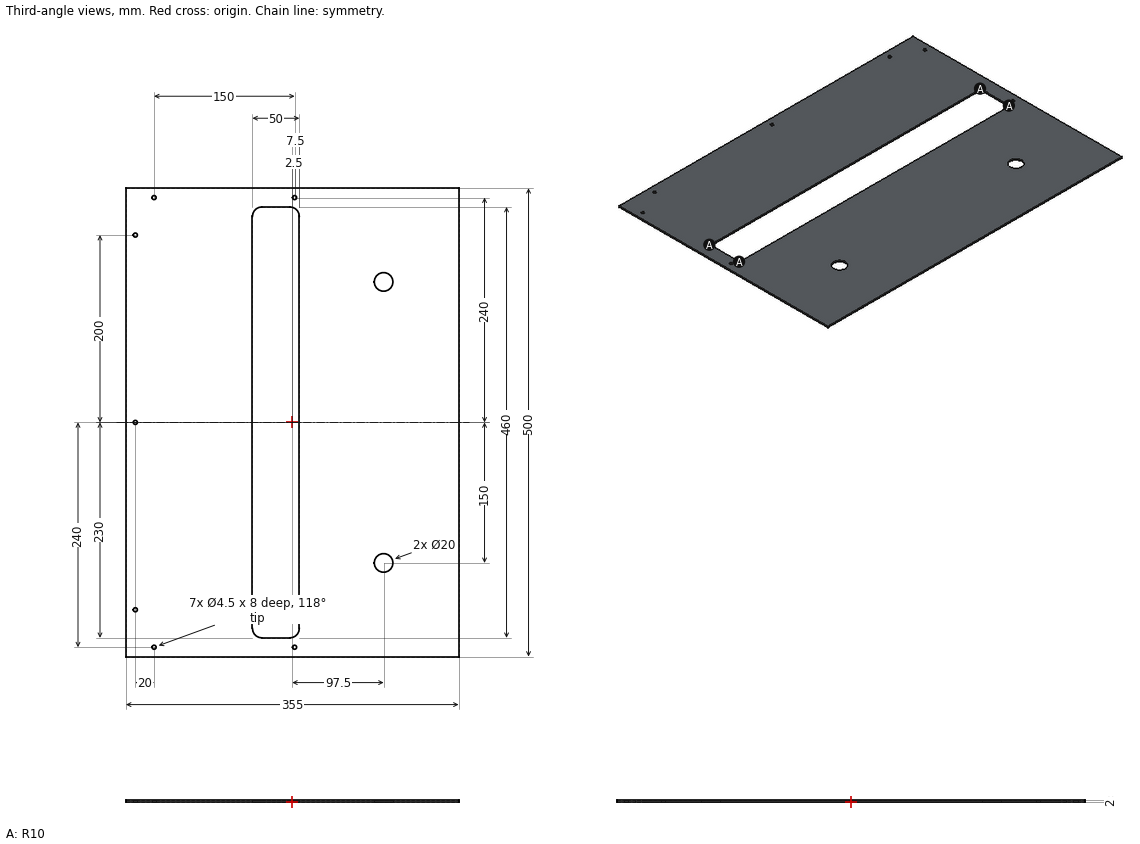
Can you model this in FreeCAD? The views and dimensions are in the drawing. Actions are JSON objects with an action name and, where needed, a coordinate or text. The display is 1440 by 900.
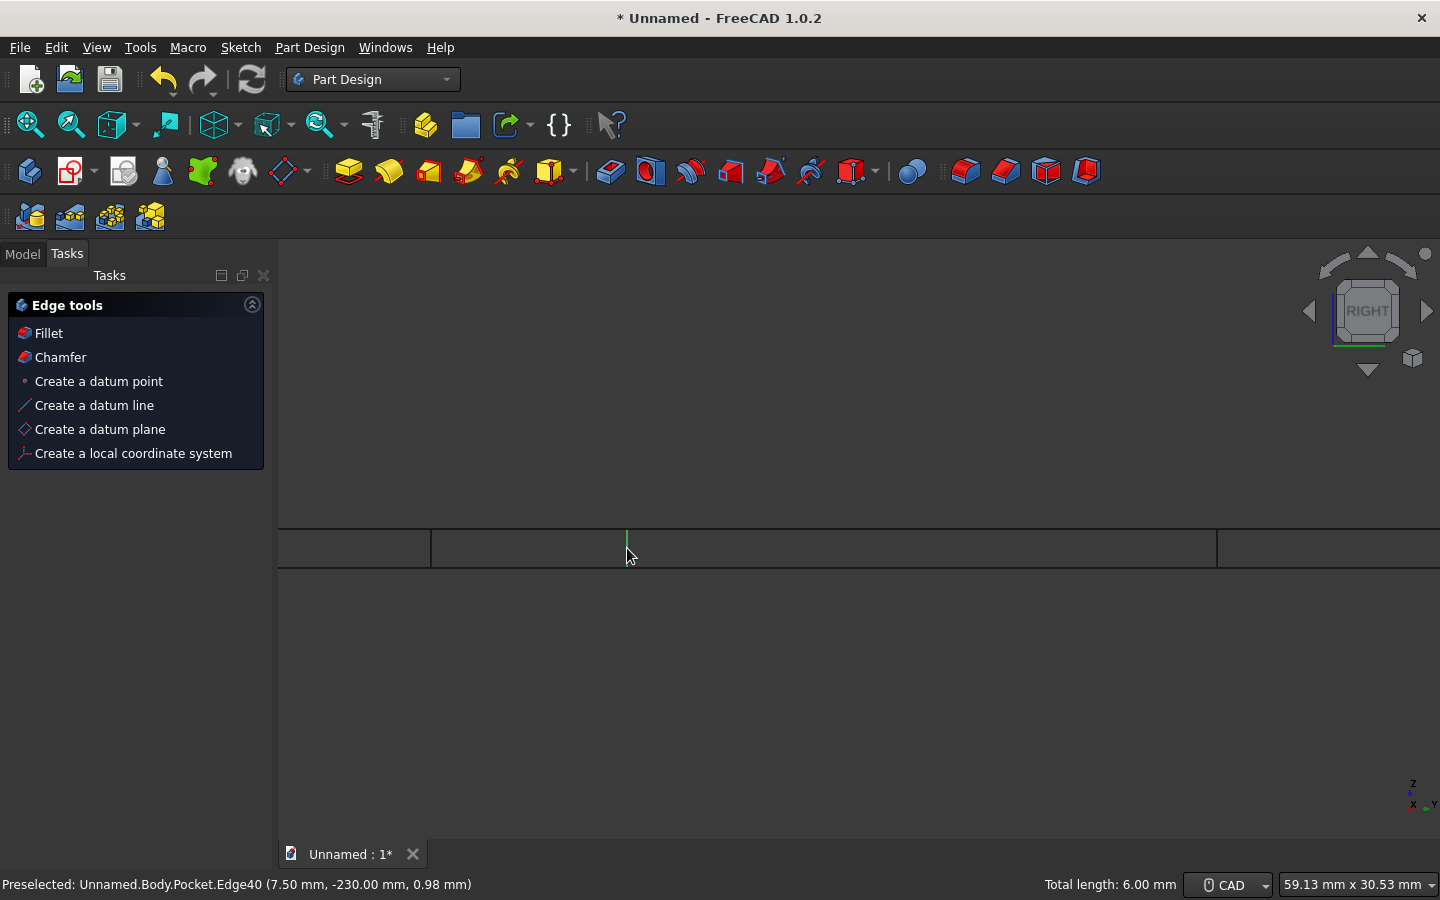
{"action": "left_click", "coordinate": [32, 126]}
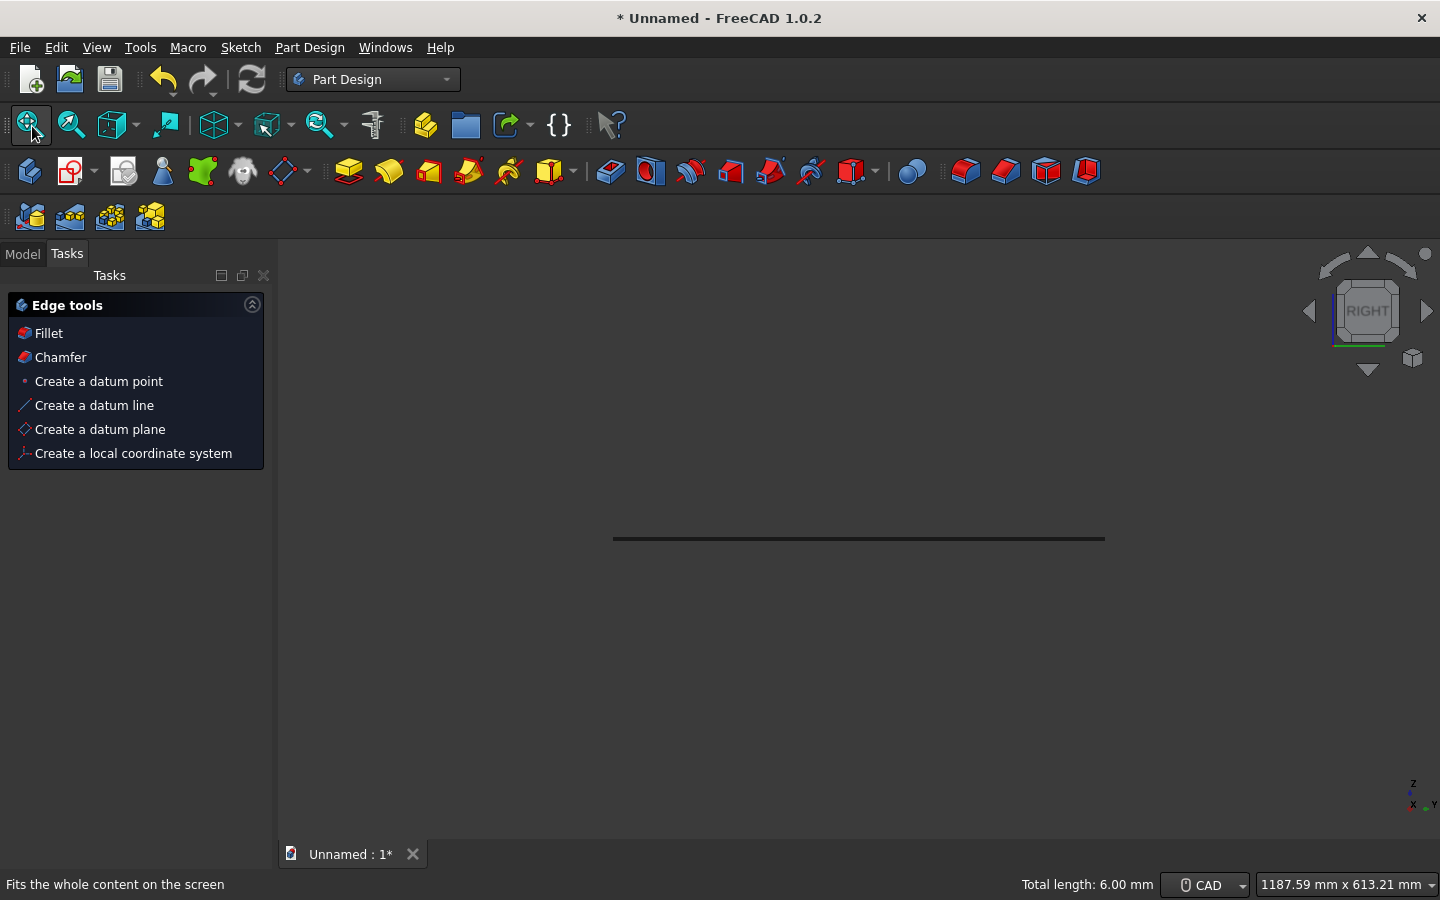
{"action": "key", "text": "5"}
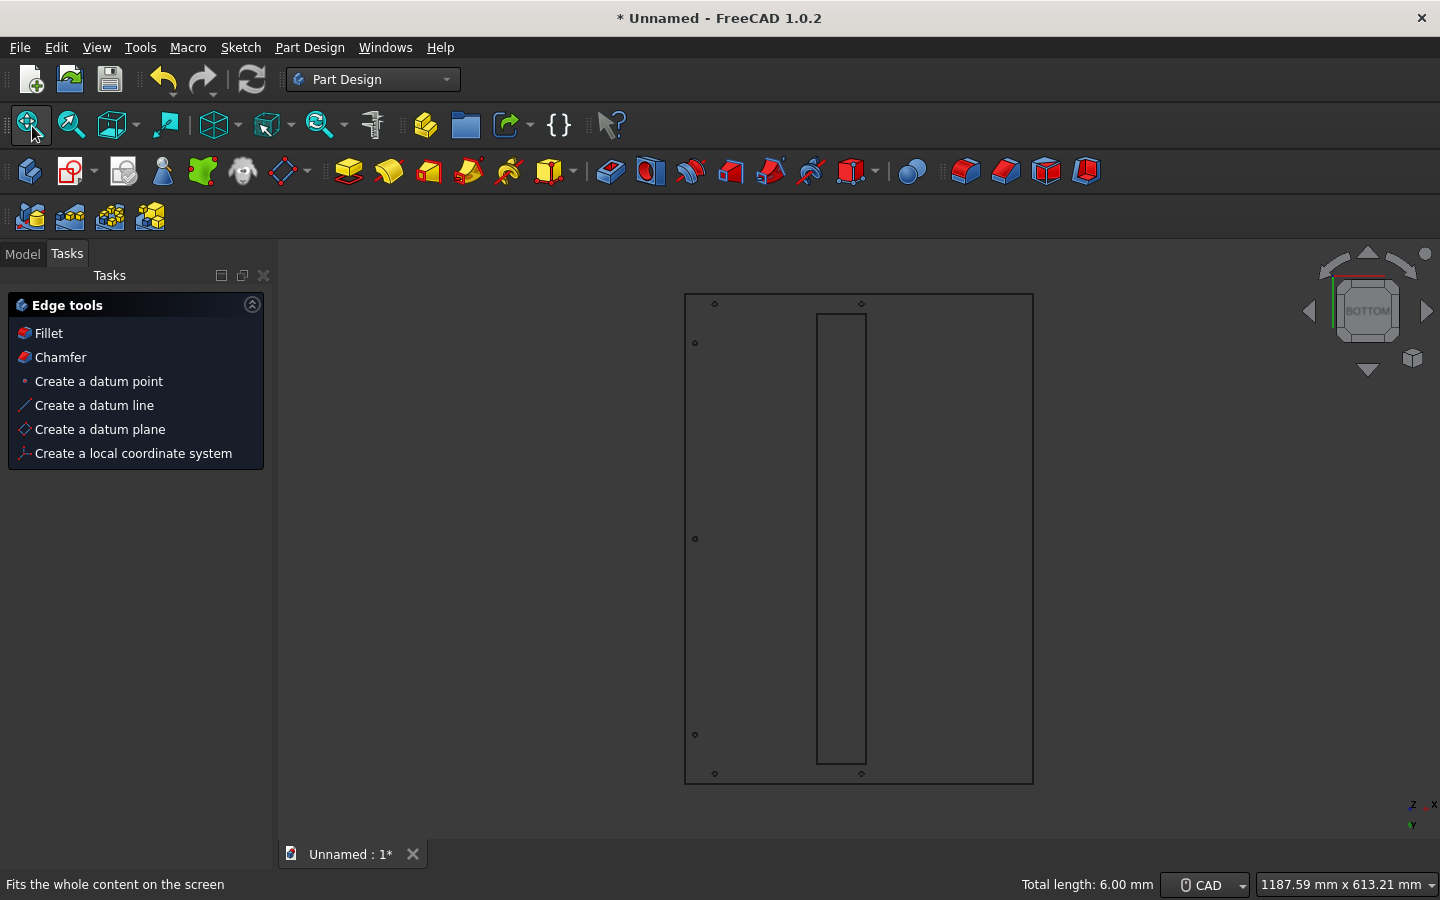
{"action": "scroll", "coordinate": [866, 763], "scroll_direction": "up", "scroll_amount": 15}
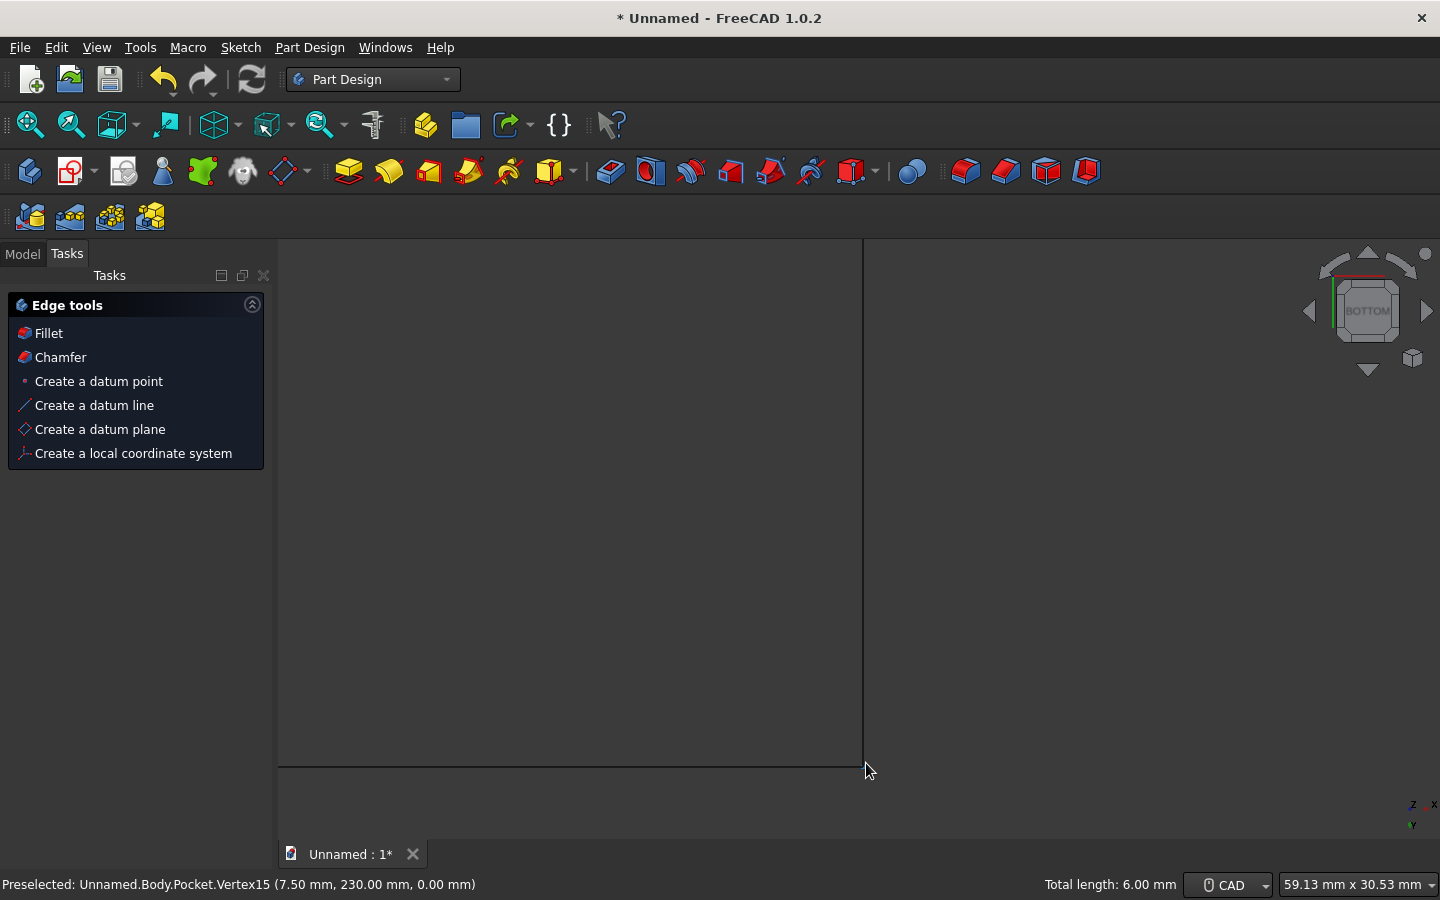
{"action": "left_click", "coordinate": [32, 126]}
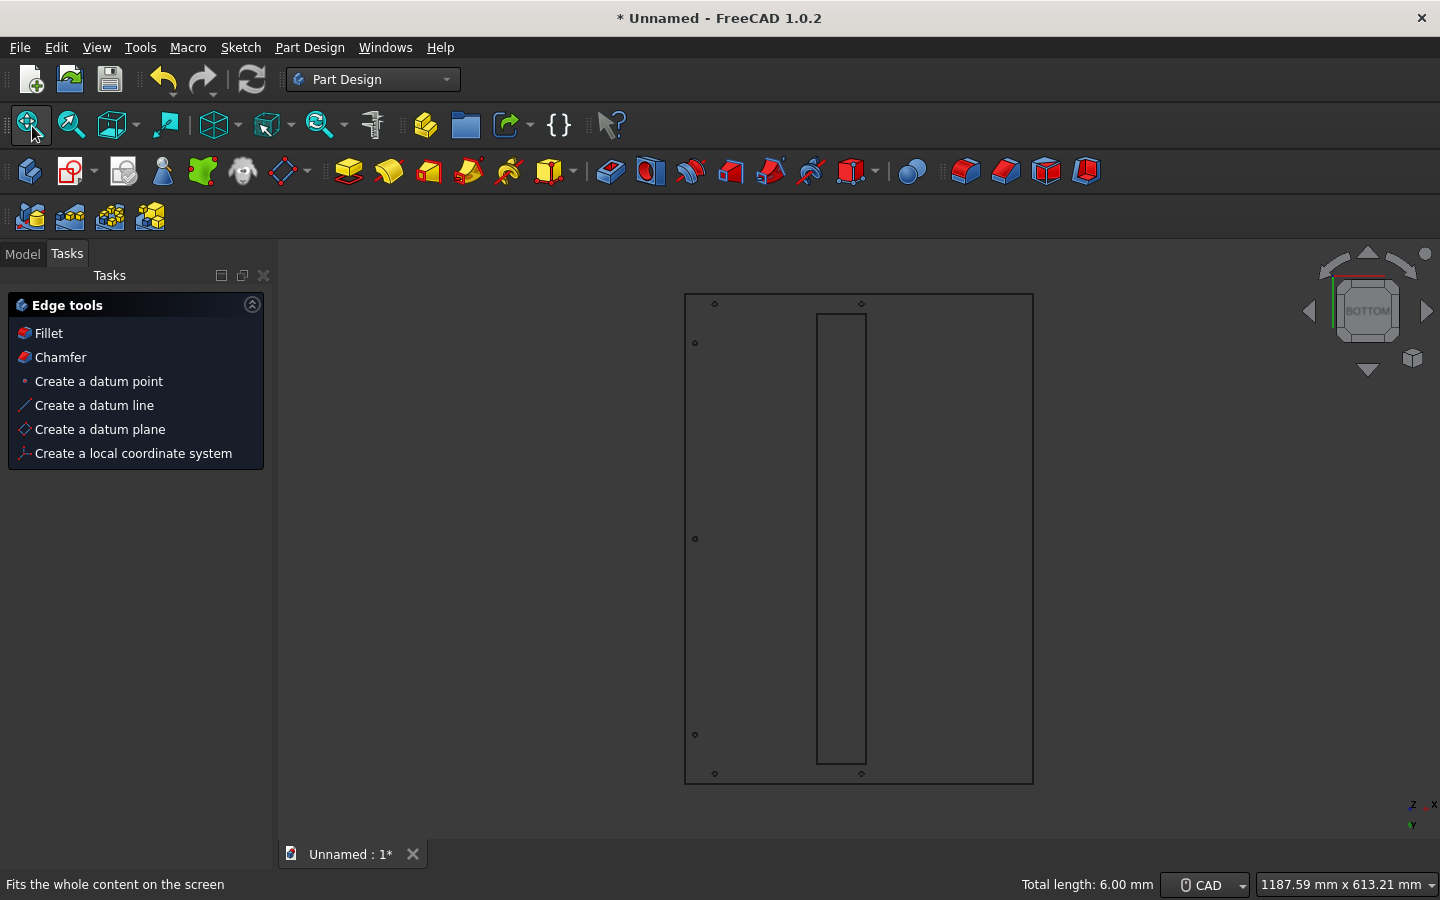
{"action": "key", "text": "4"}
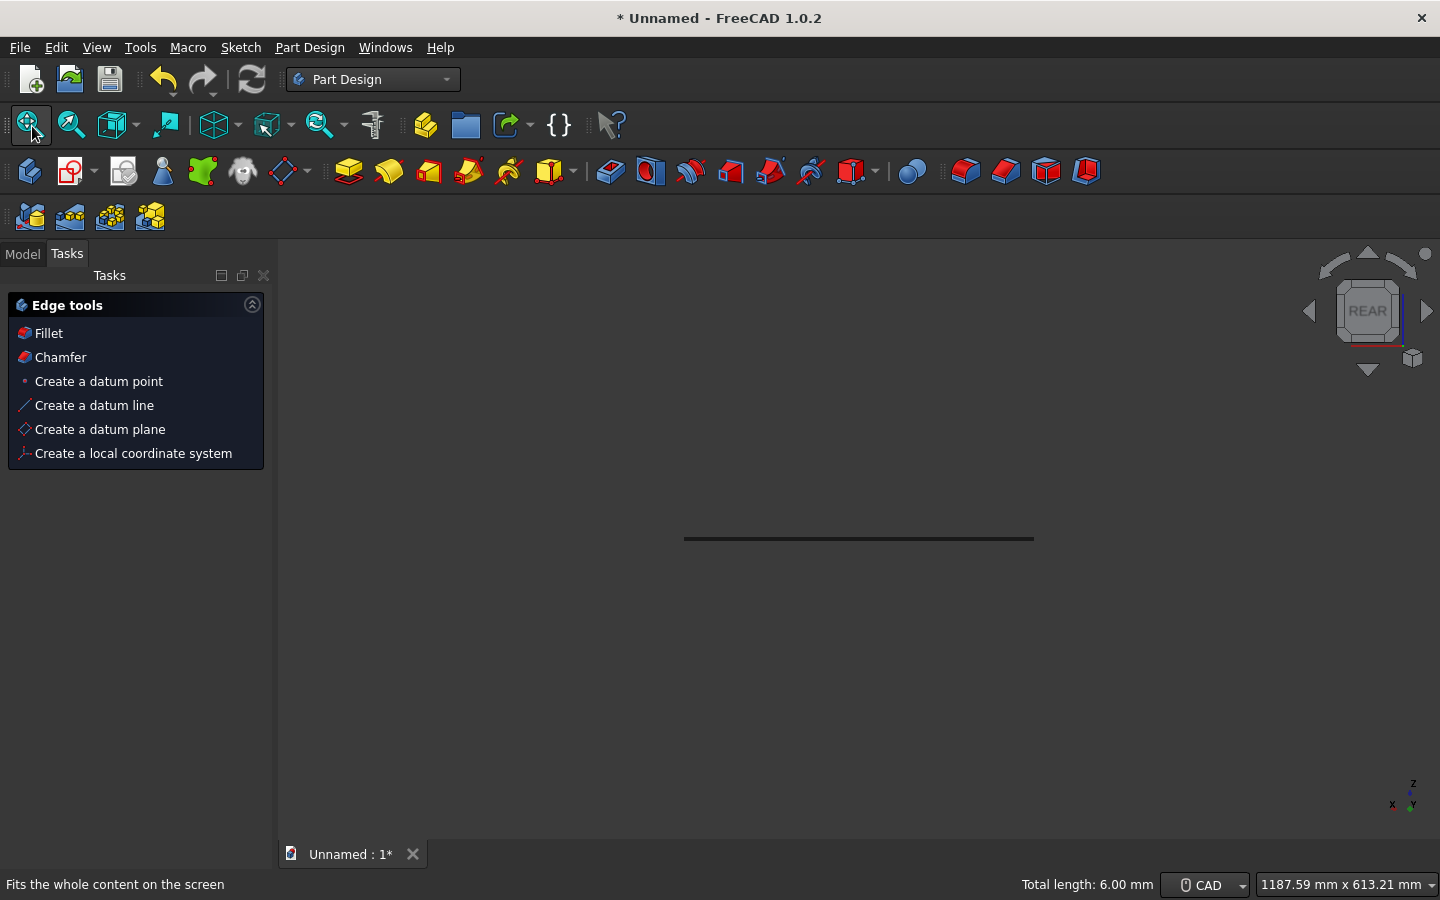
{"action": "left_click", "coordinate": [32, 126]}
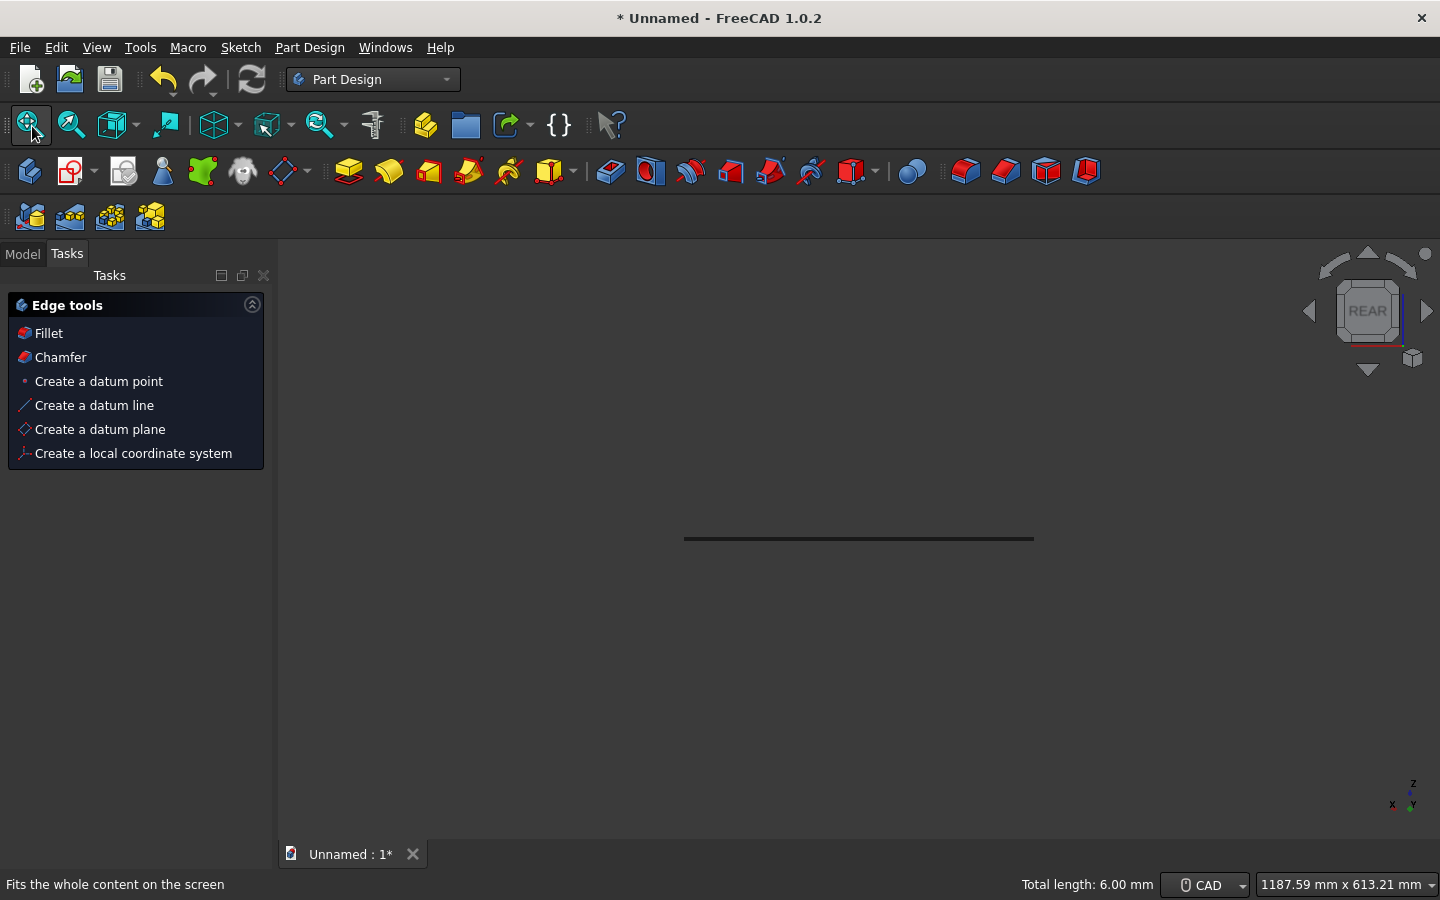
{"action": "scroll", "coordinate": [852, 538], "scroll_direction": "up", "scroll_amount": 15}